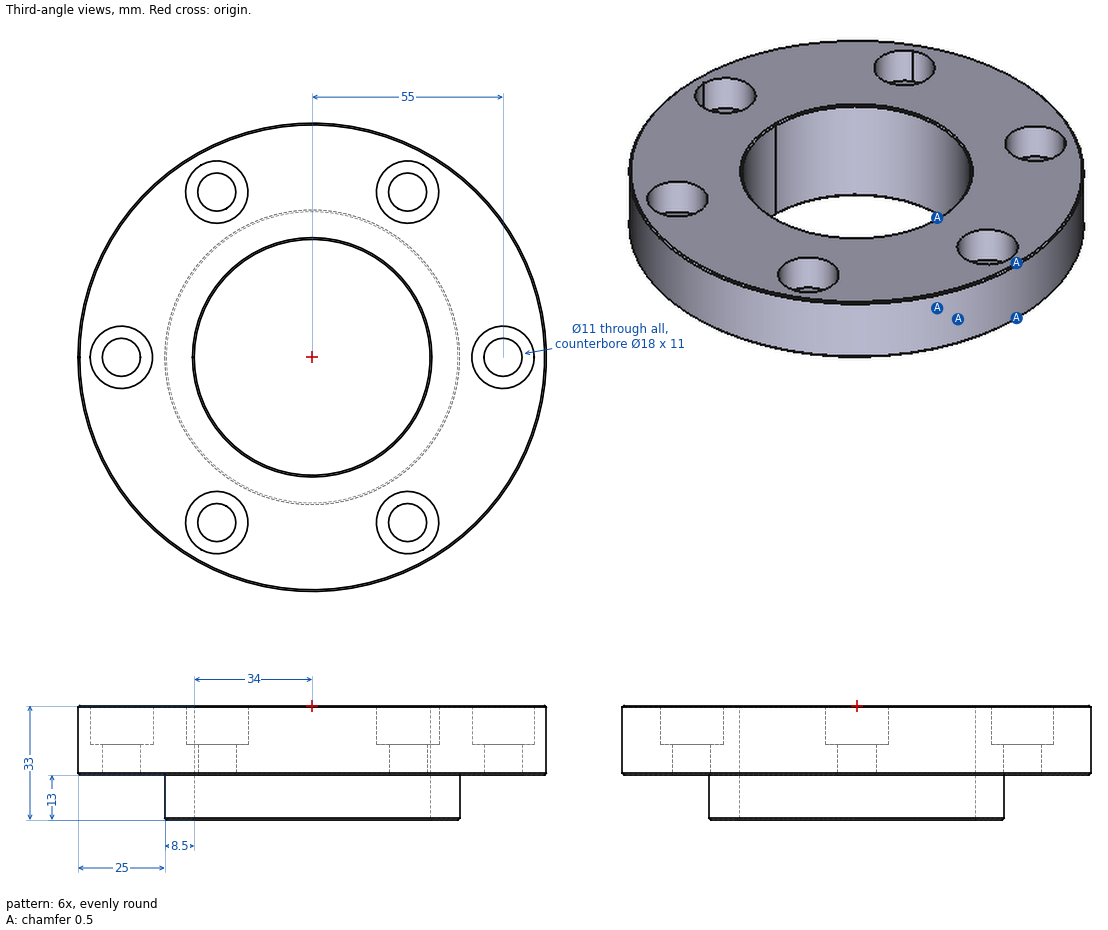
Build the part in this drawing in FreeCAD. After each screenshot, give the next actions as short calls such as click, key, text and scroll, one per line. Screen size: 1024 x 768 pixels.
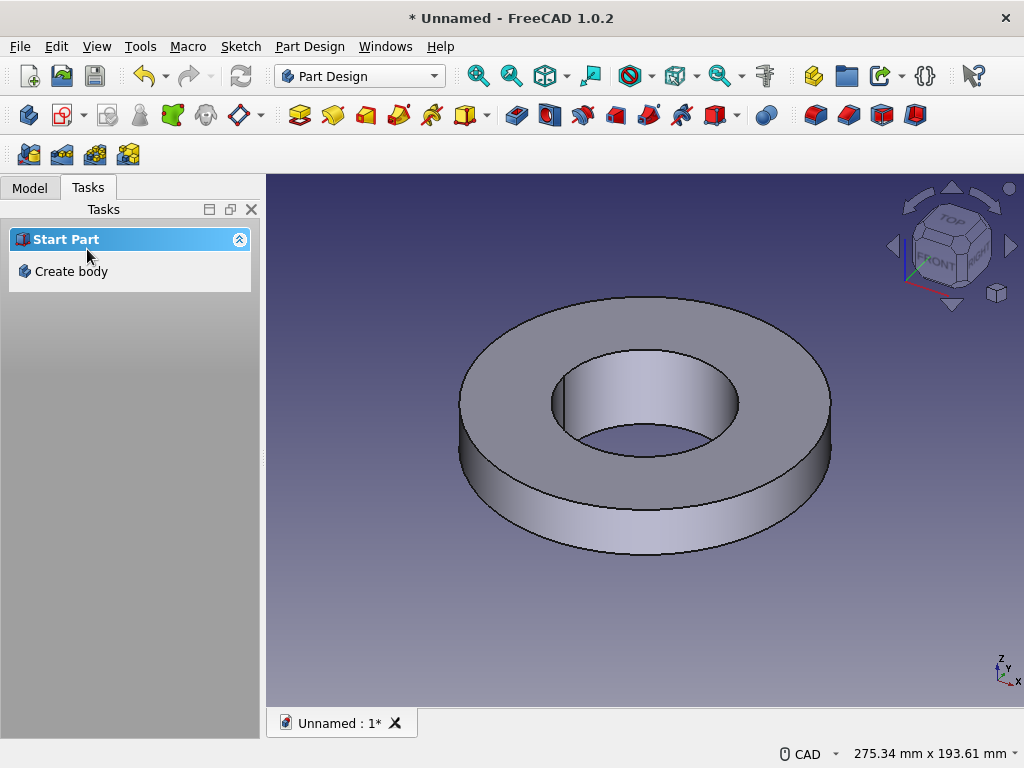
click(62, 116)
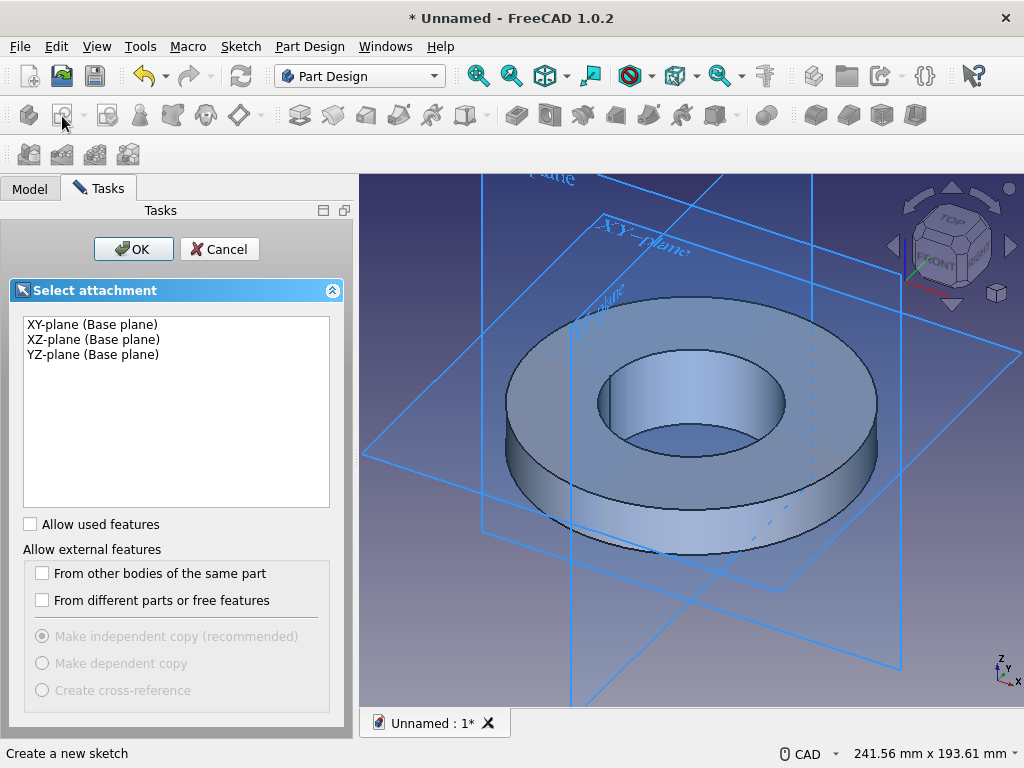
click(84, 324)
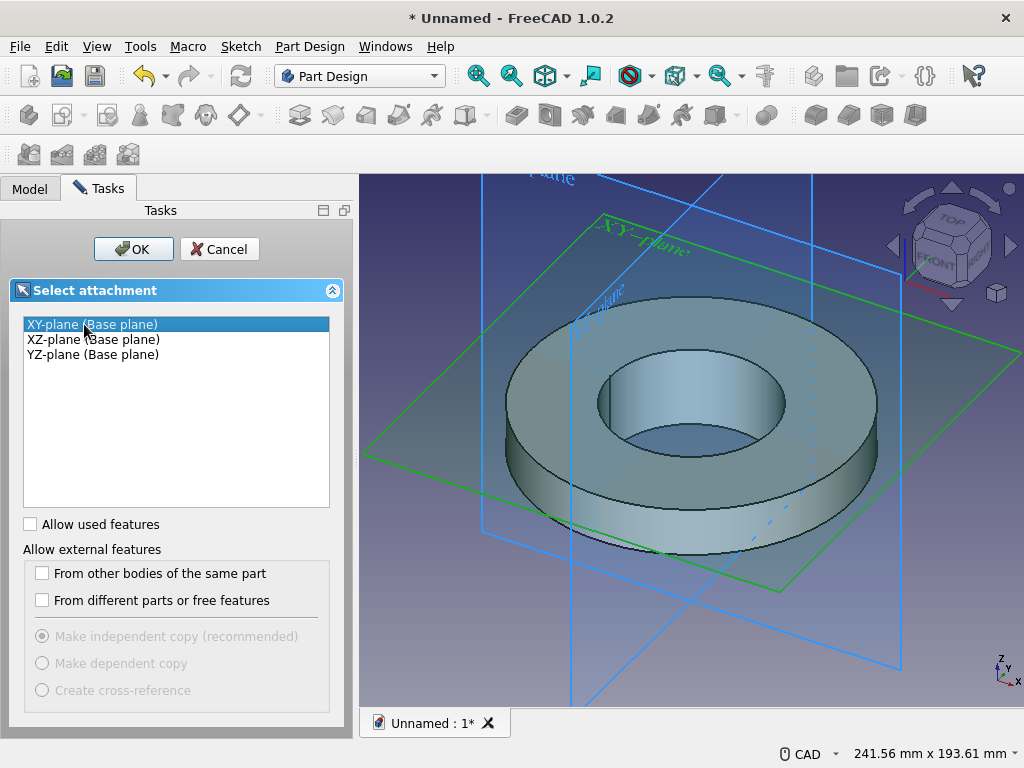
click(134, 249)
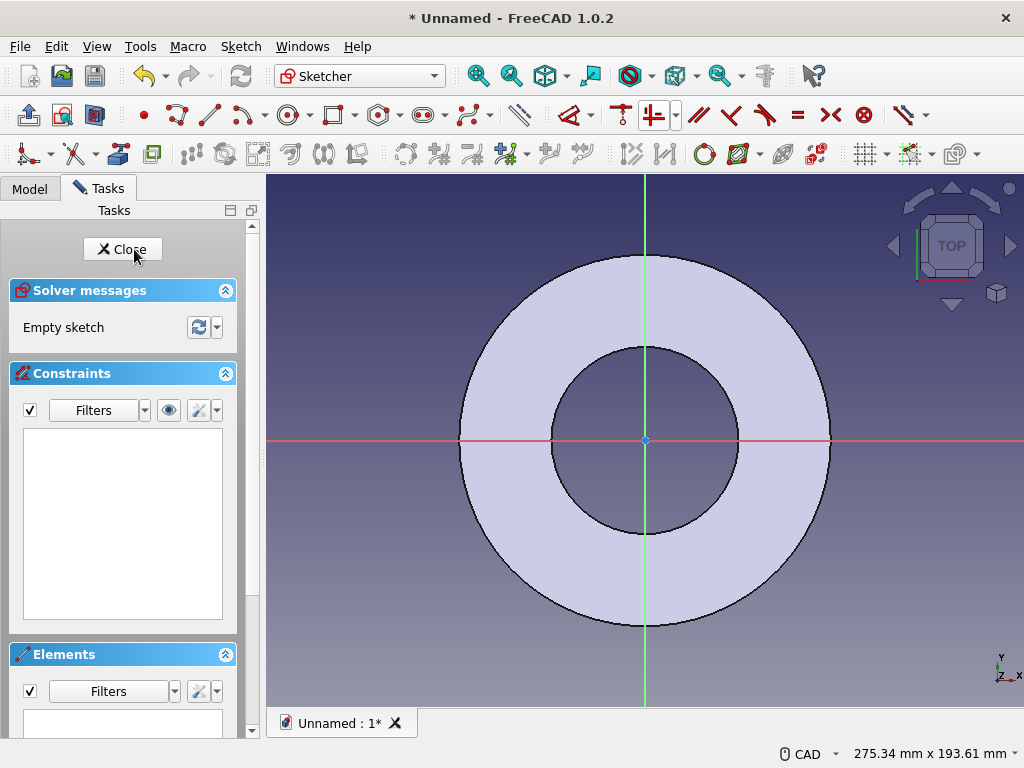
scroll(818, 440, up, 12)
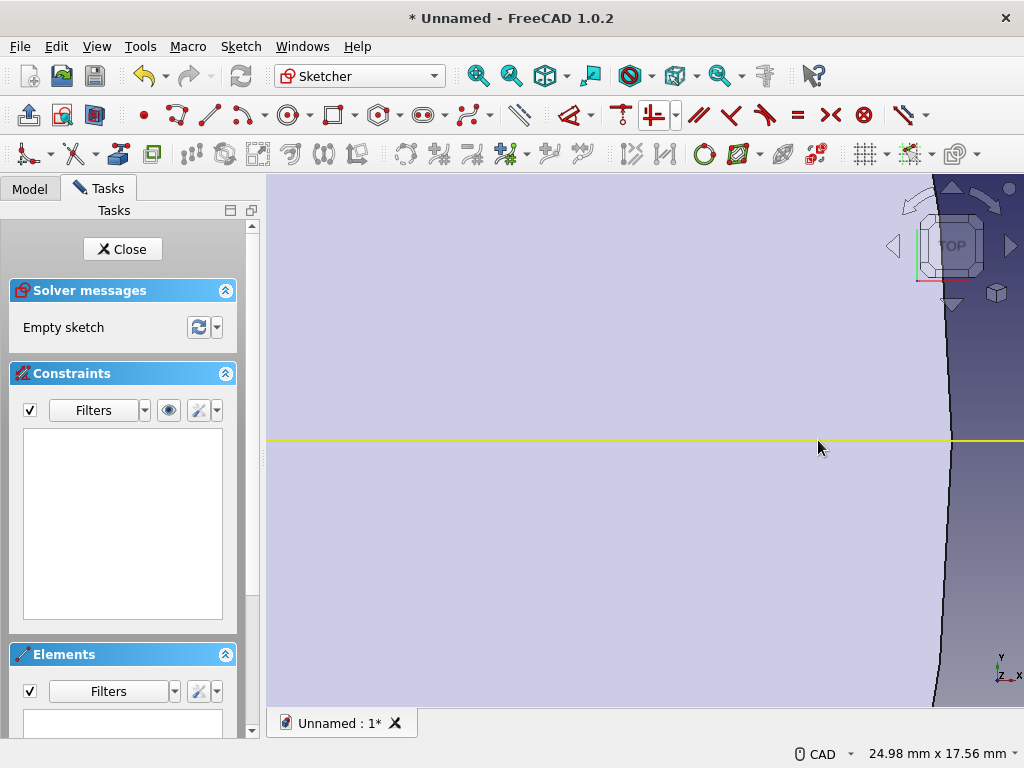
click(288, 116)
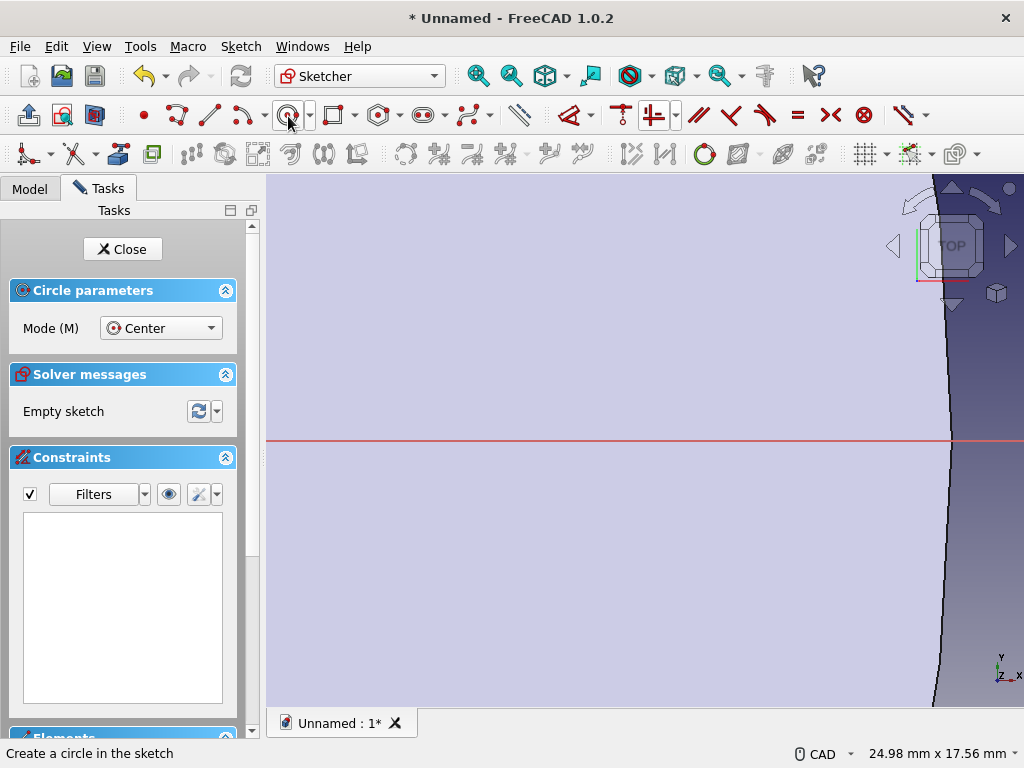
click(573, 440)
move(691, 322)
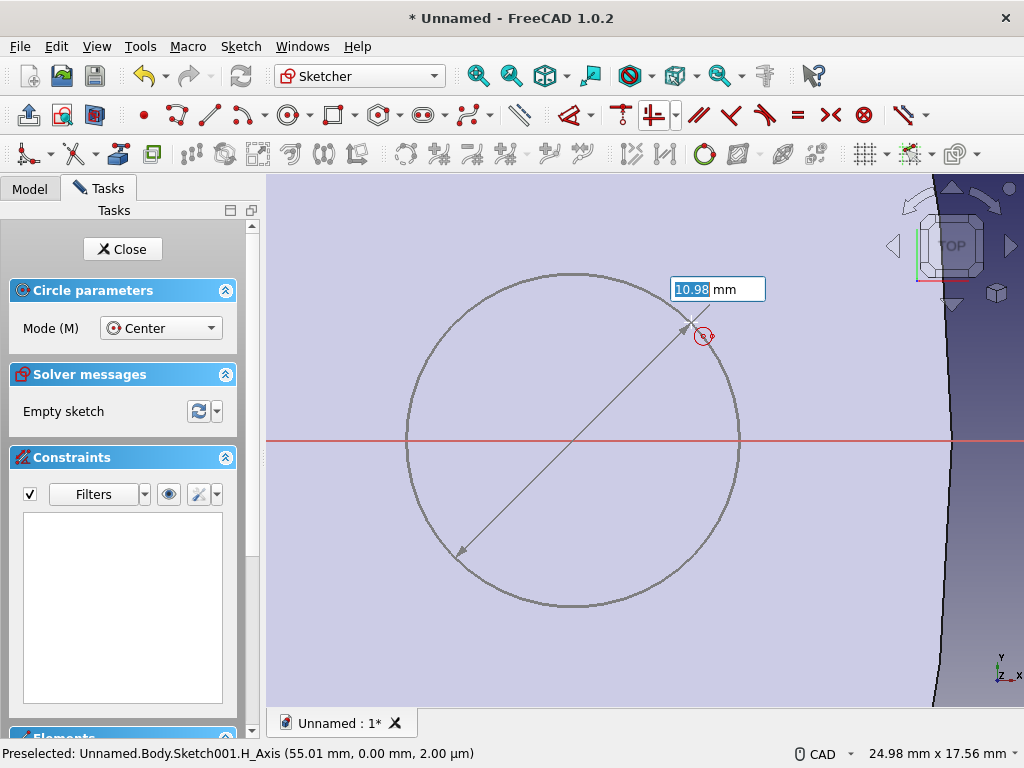
text(11)
key(Return)
key(Escape)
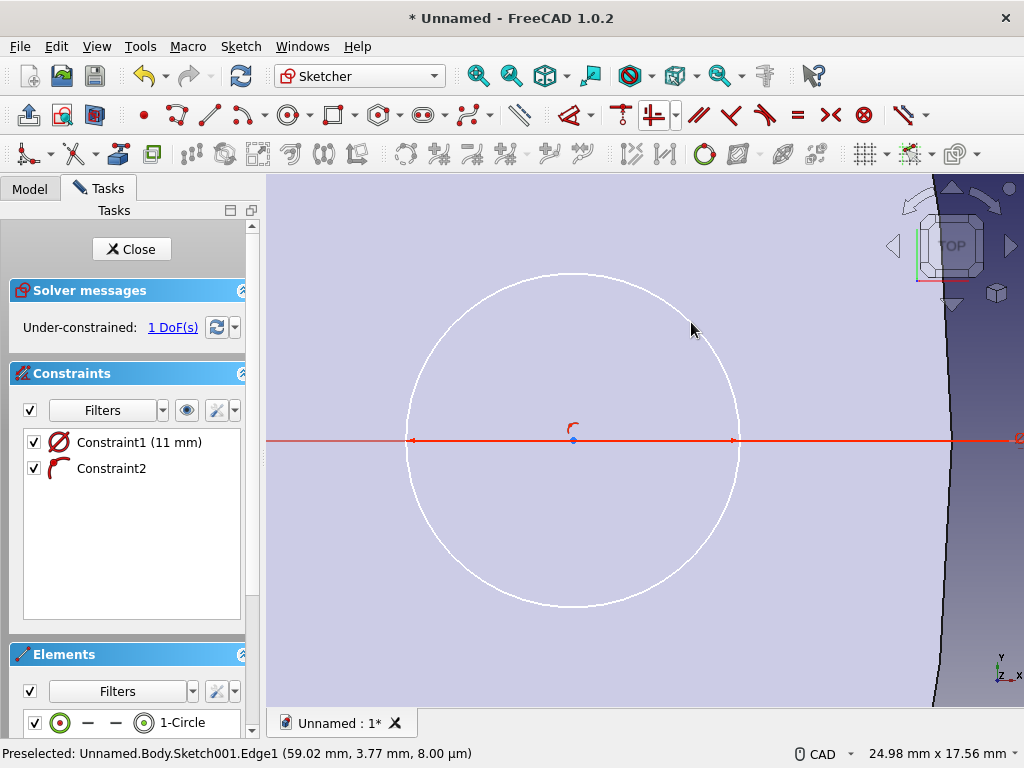
click(568, 116)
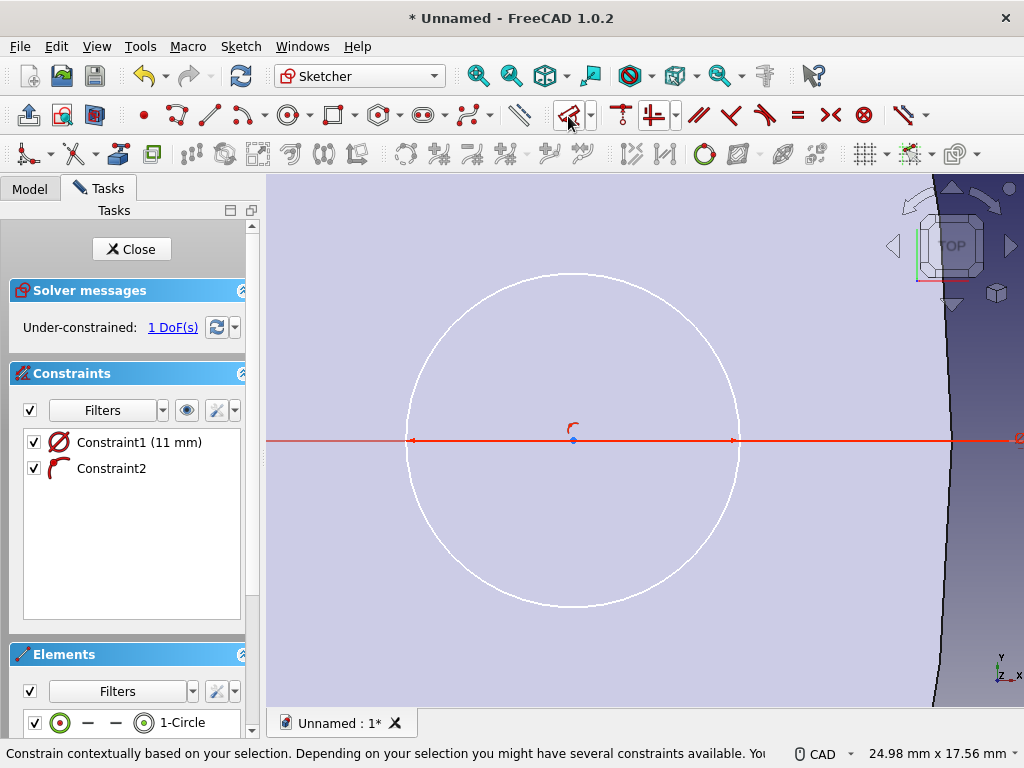
click(573, 440)
click(433, 474)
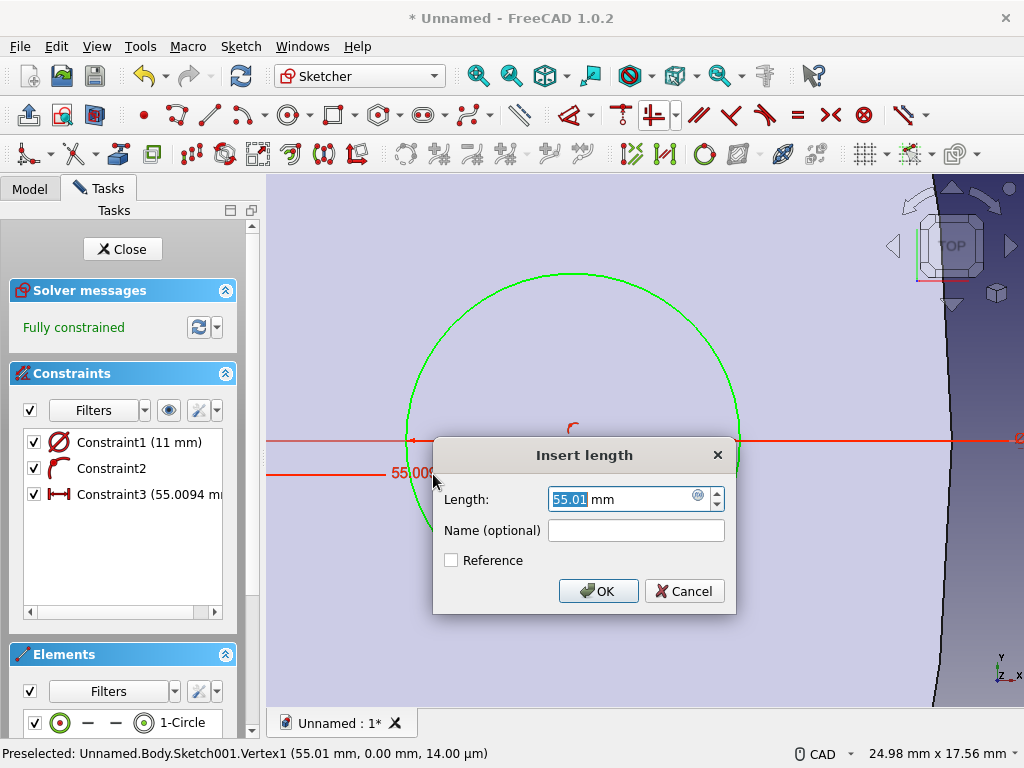
text(55)
key(Return)
key(Escape)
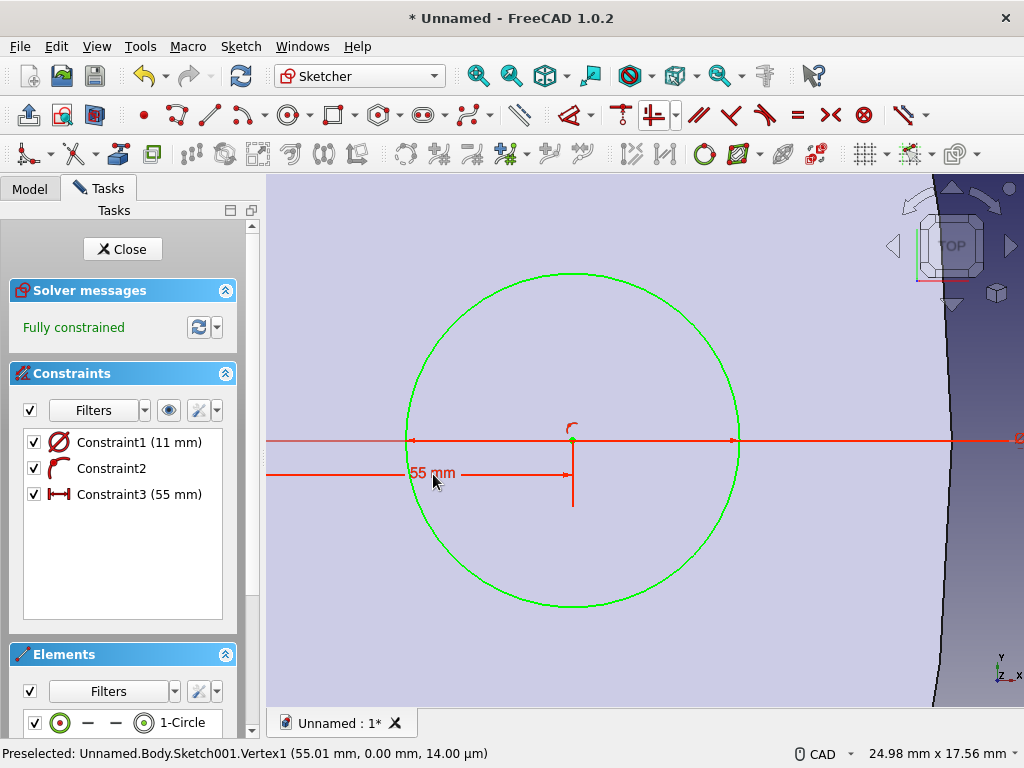
click(123, 249)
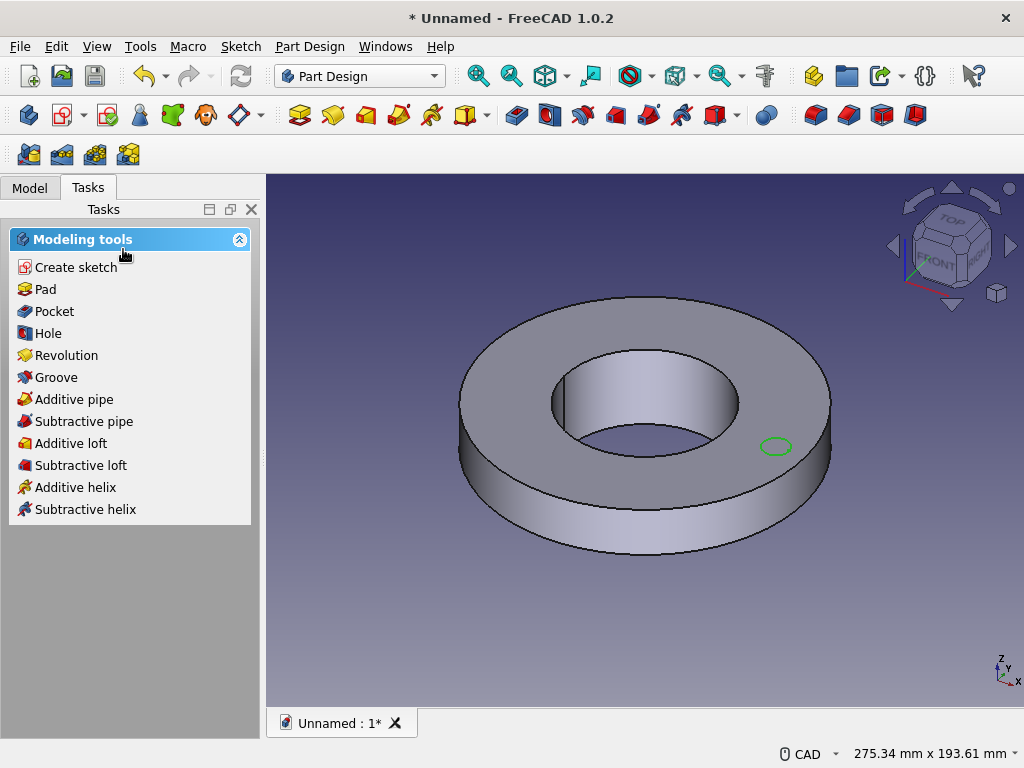
click(550, 116)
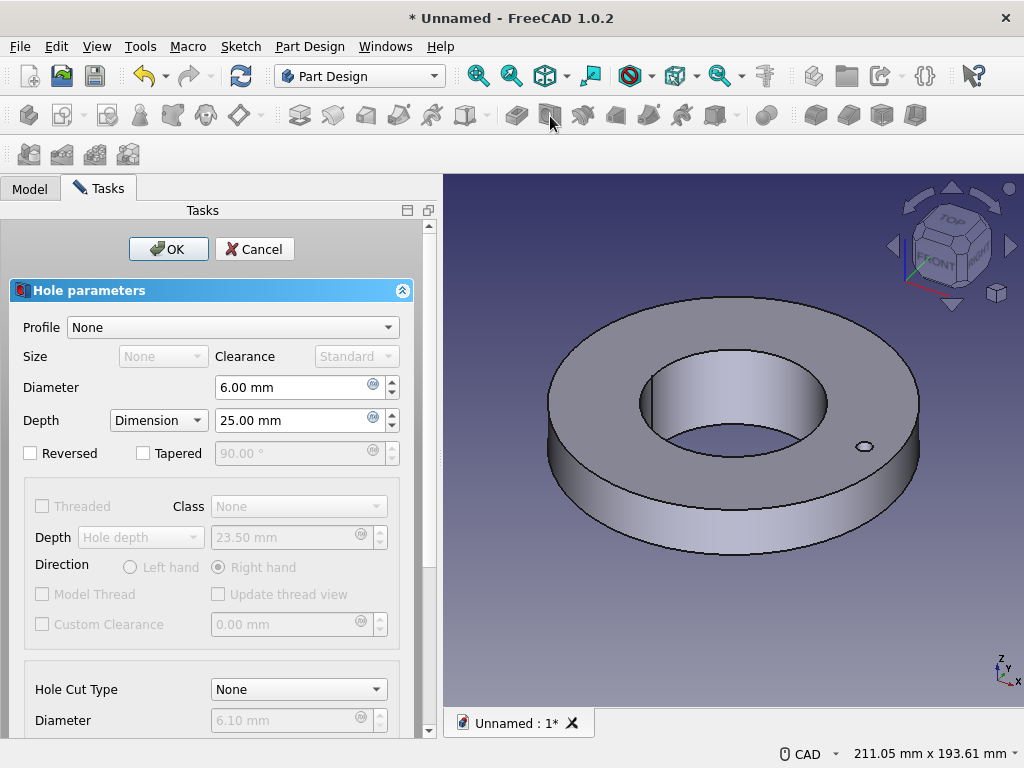
triple_click(300, 388)